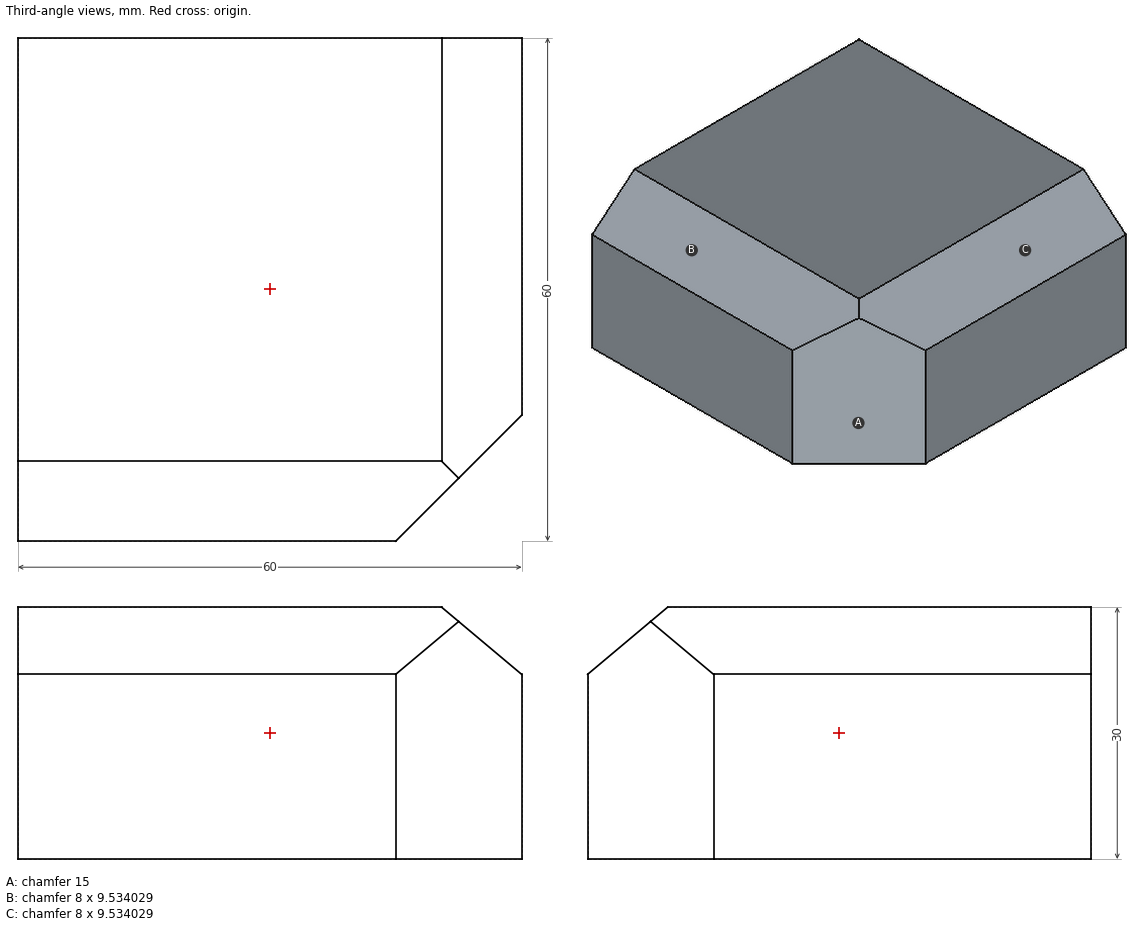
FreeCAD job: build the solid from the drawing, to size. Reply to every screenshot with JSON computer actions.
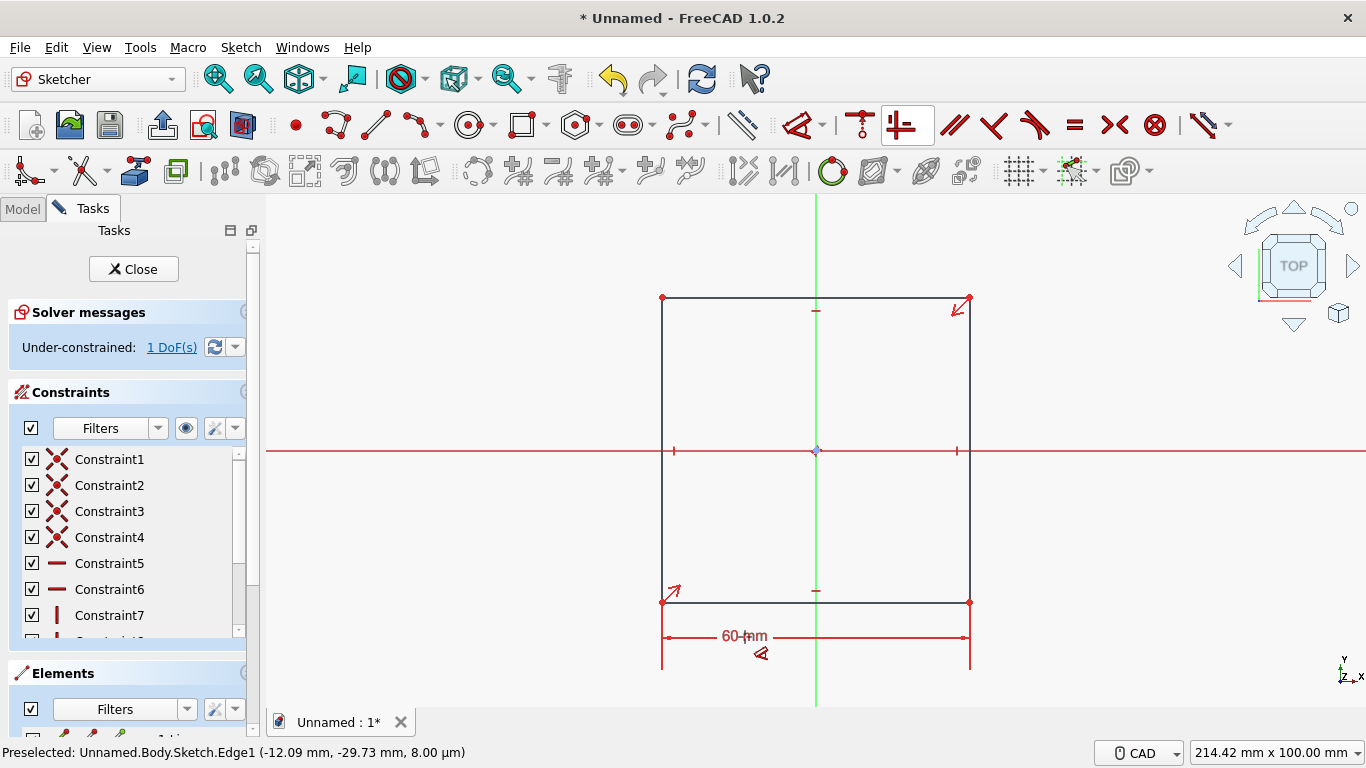
{"action": "left_click", "coordinate": [970, 511]}
{"action": "left_click", "coordinate": [1004, 380]}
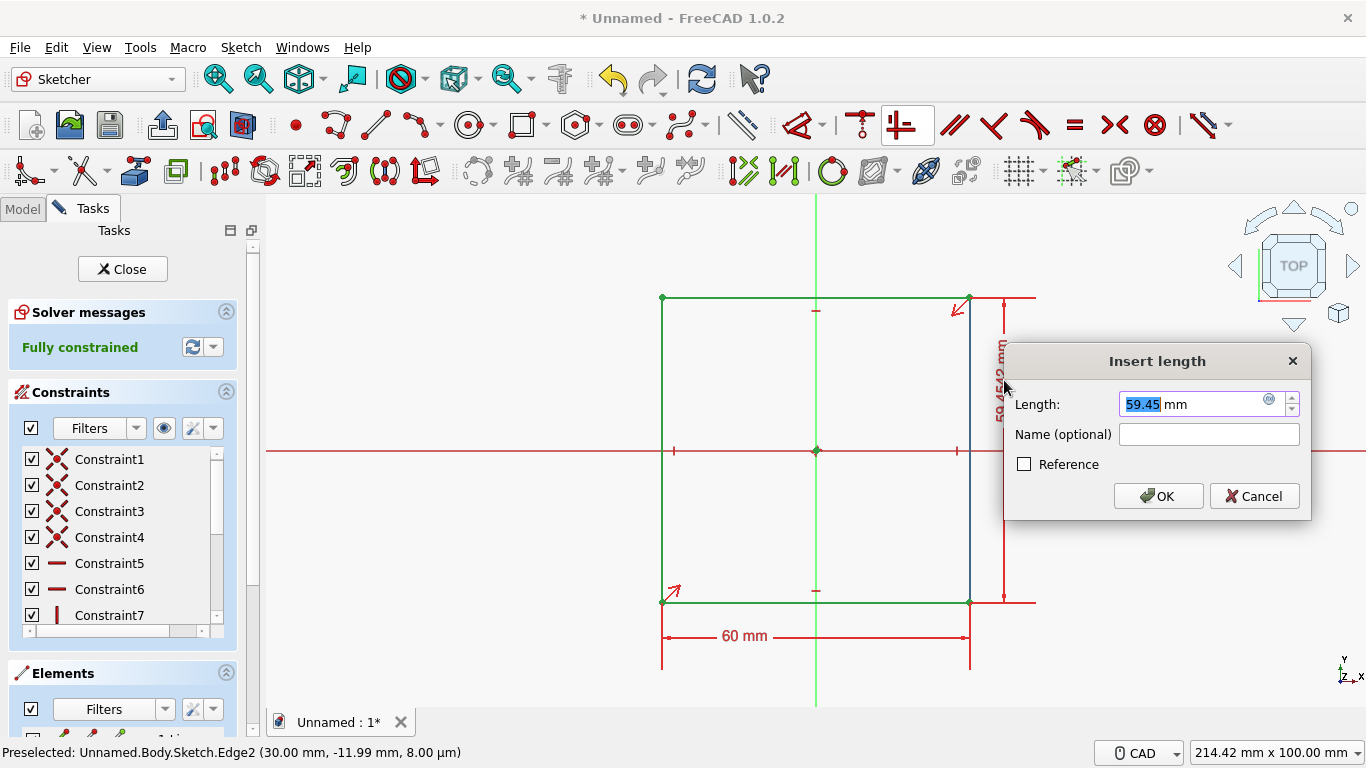
{"action": "type", "text": "60"}
{"action": "key", "text": "Return"}
{"action": "key", "text": "Escape"}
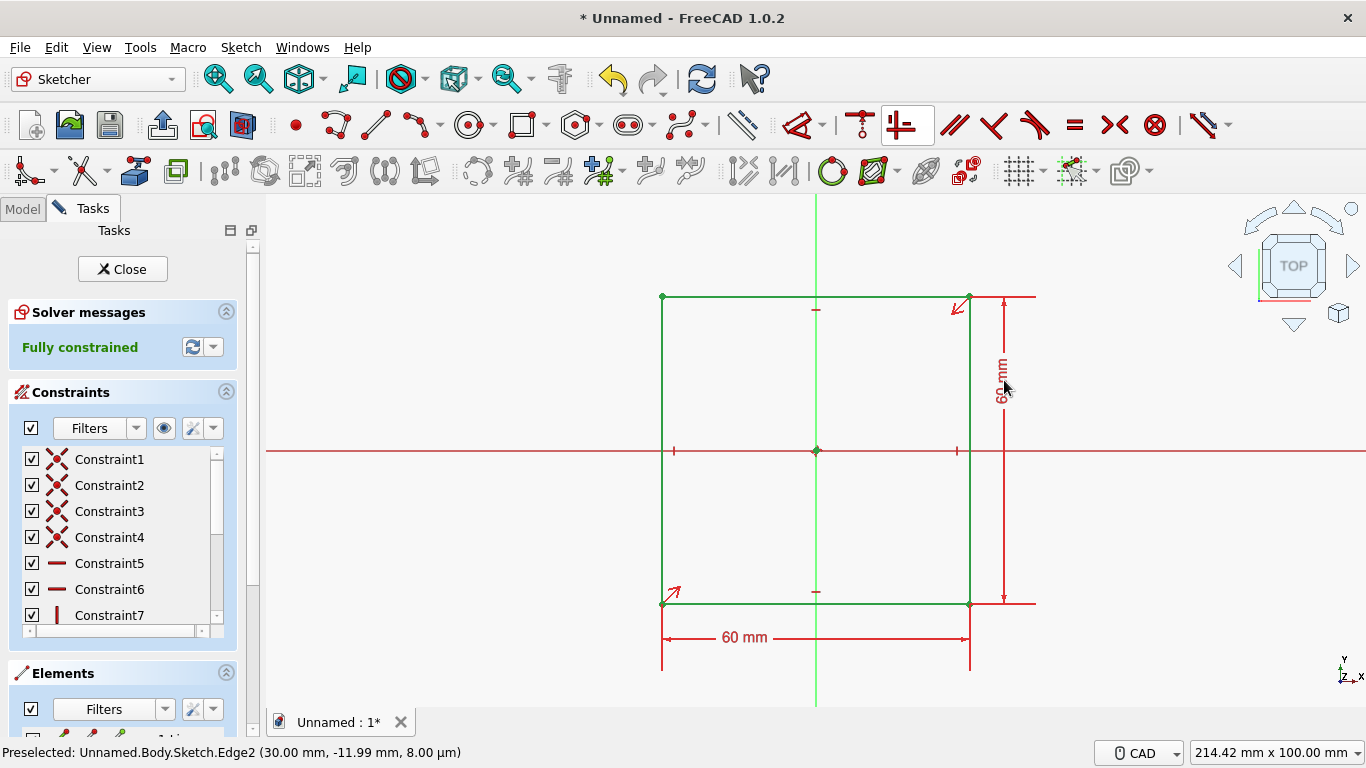
{"action": "left_click", "coordinate": [123, 269]}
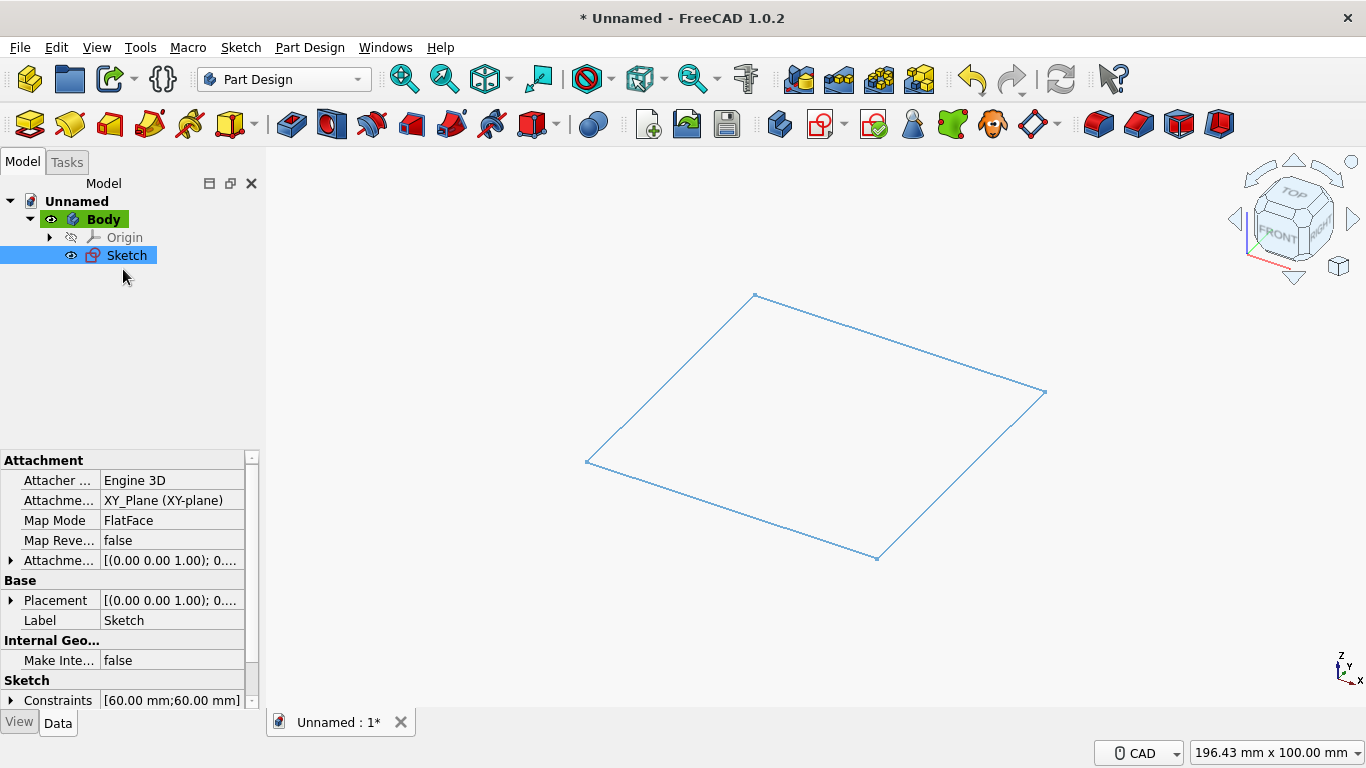
{"action": "left_click", "coordinate": [30, 124]}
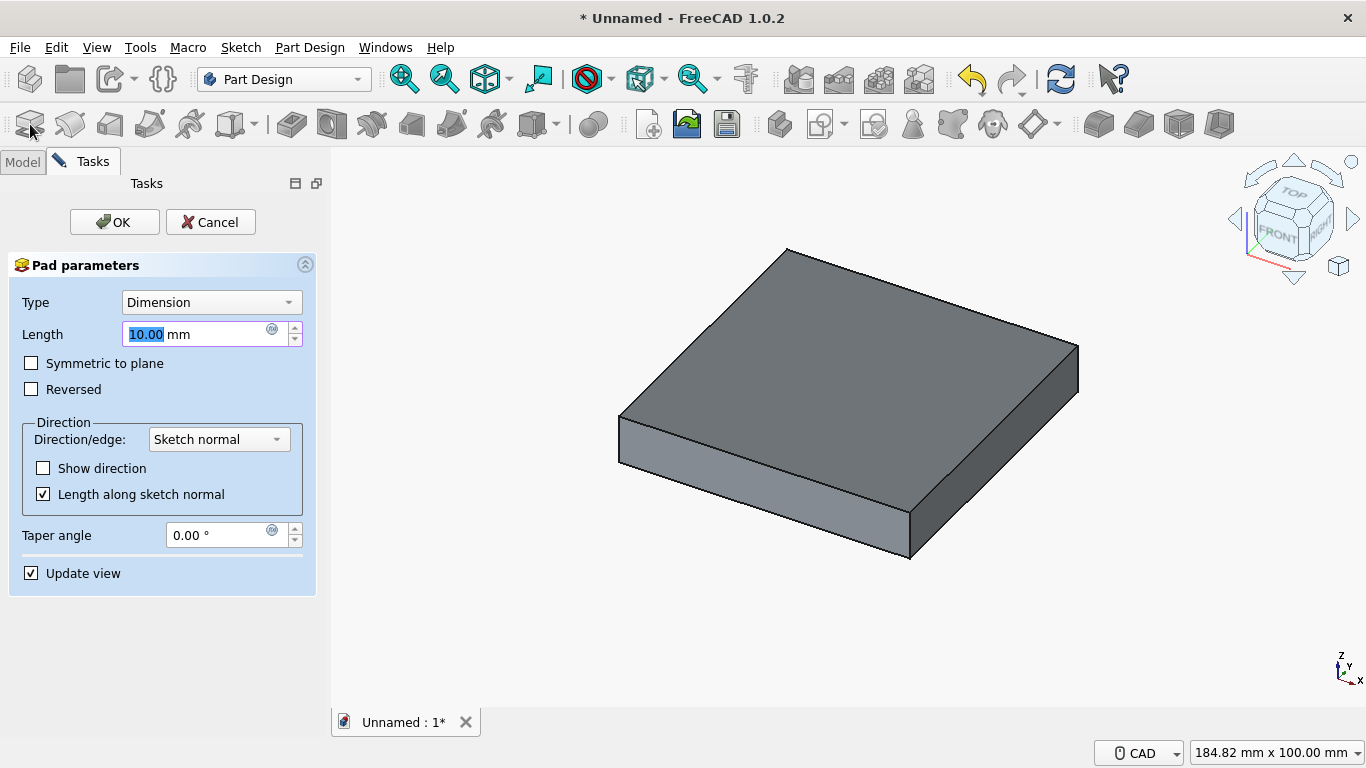
{"action": "type", "text": "30"}
{"action": "key", "text": "Tab"}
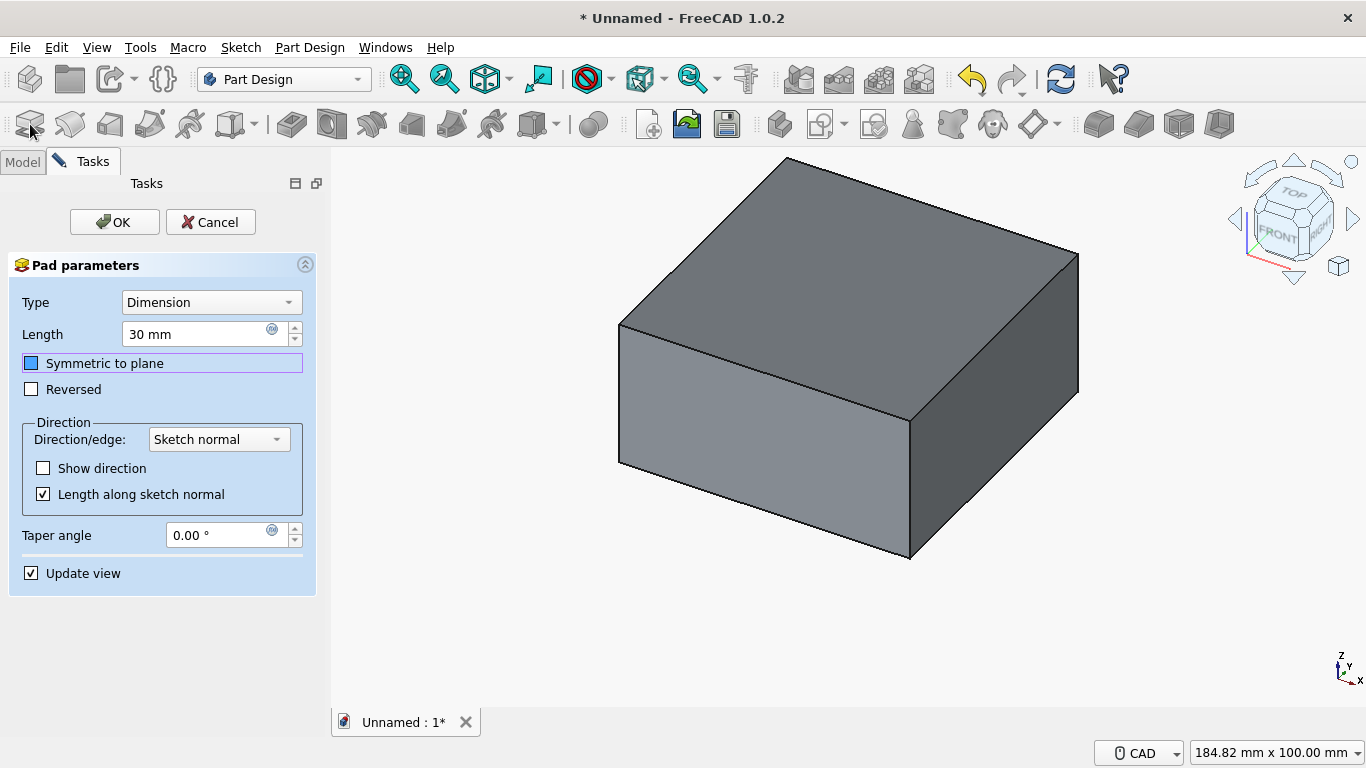
{"action": "left_click", "coordinate": [30, 363]}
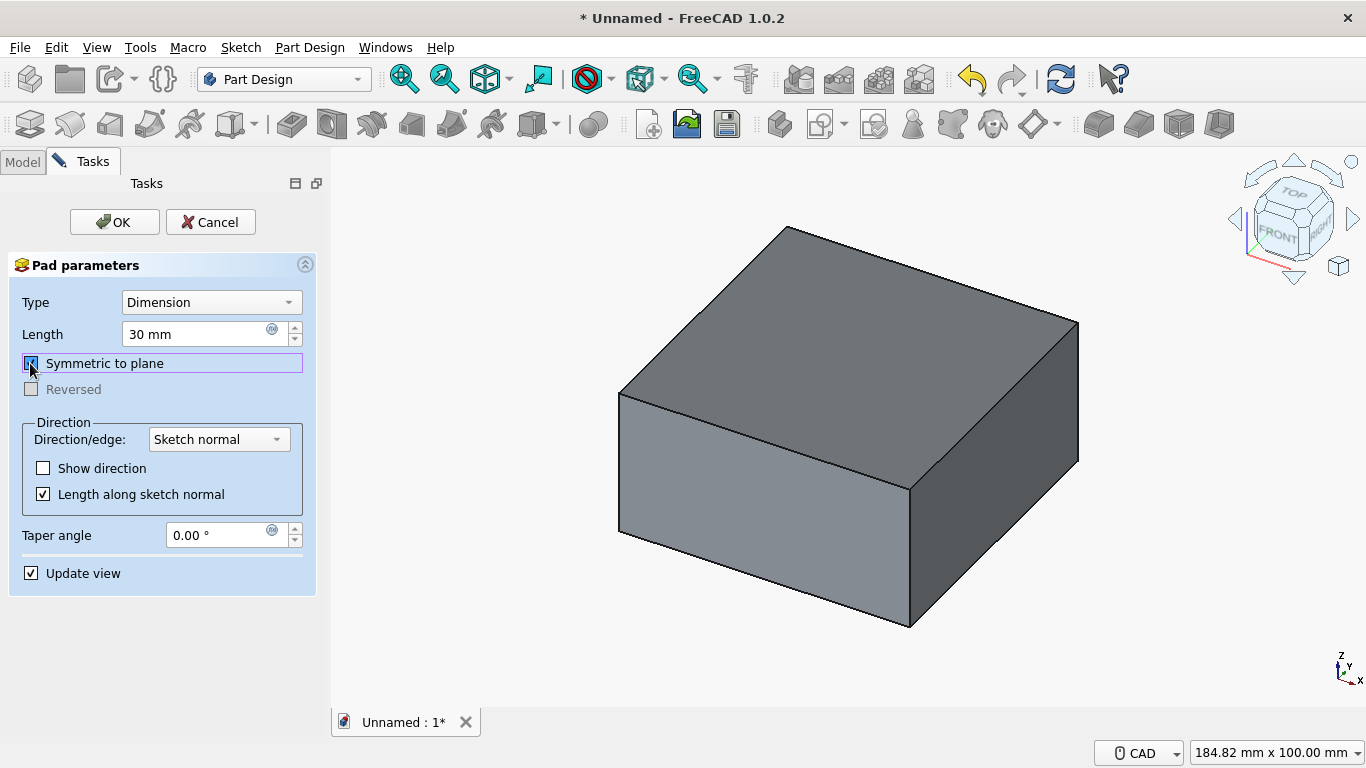
{"action": "left_click", "coordinate": [115, 222]}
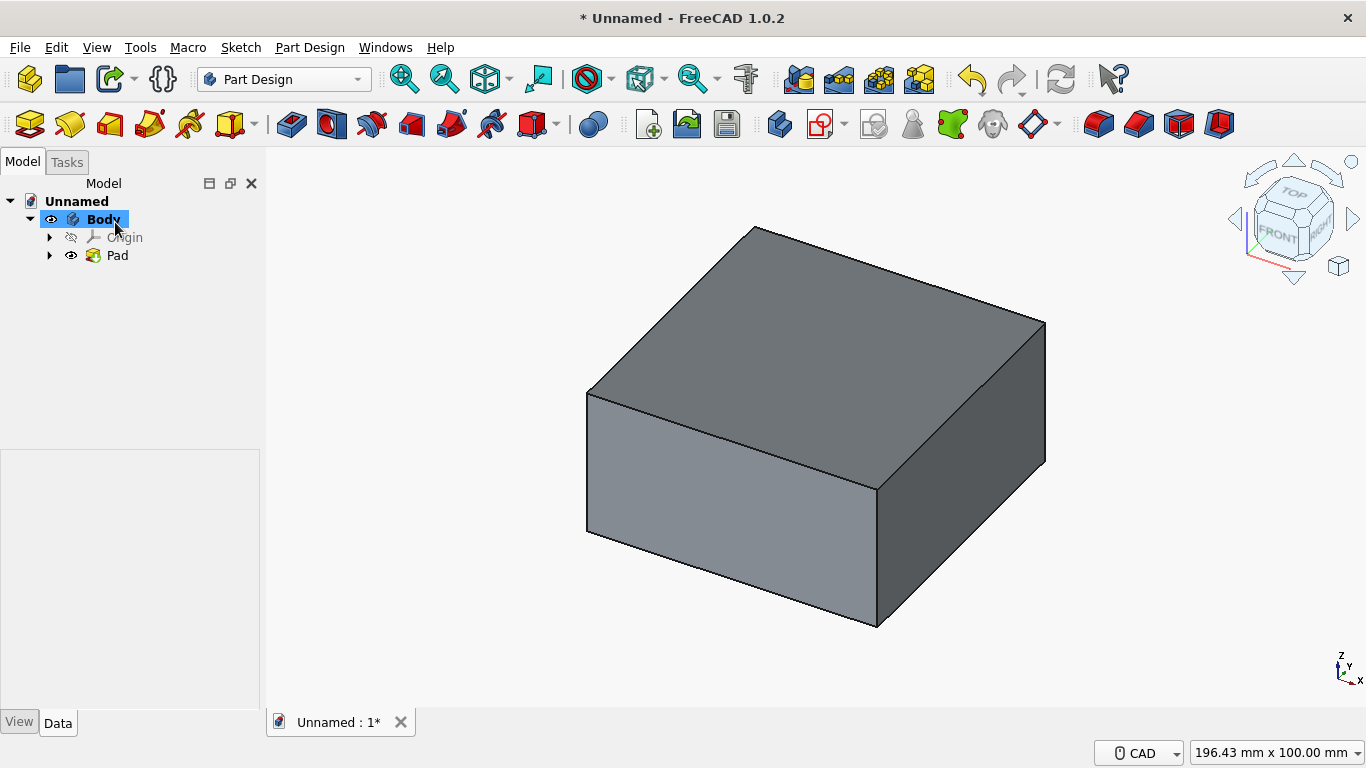
{"action": "left_click", "coordinate": [877, 558]}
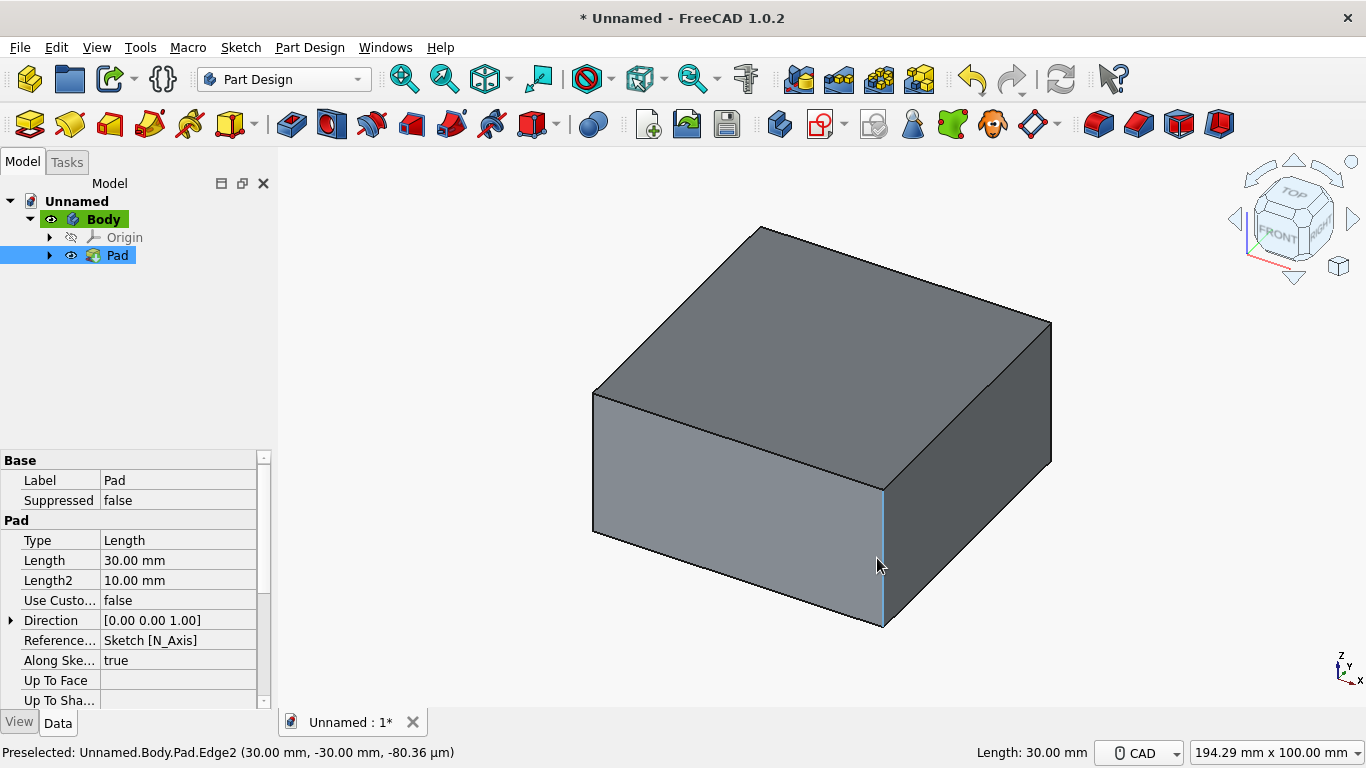
{"action": "left_click", "coordinate": [1140, 124]}